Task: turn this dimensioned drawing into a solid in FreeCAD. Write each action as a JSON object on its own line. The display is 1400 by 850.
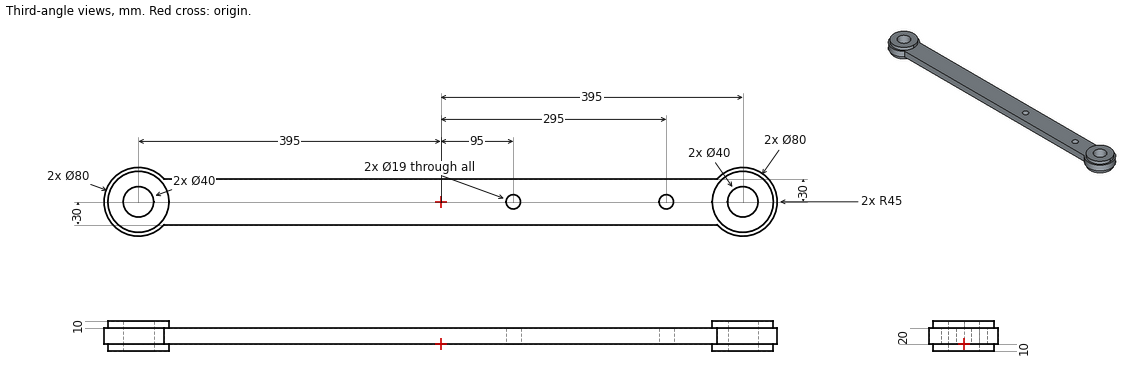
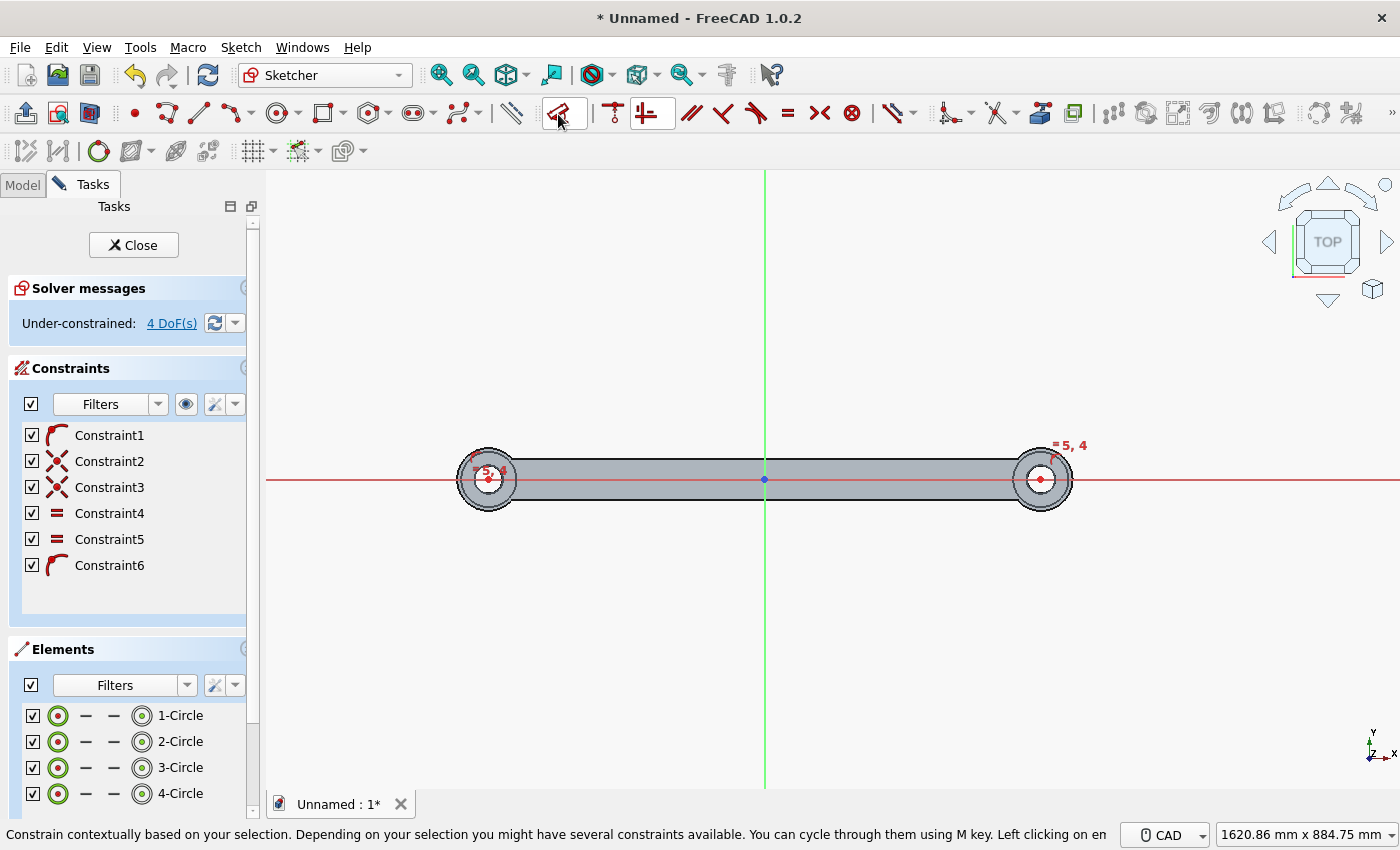
{"action": "left_click", "coordinate": [508, 460]}
{"action": "left_click", "coordinate": [530, 437]}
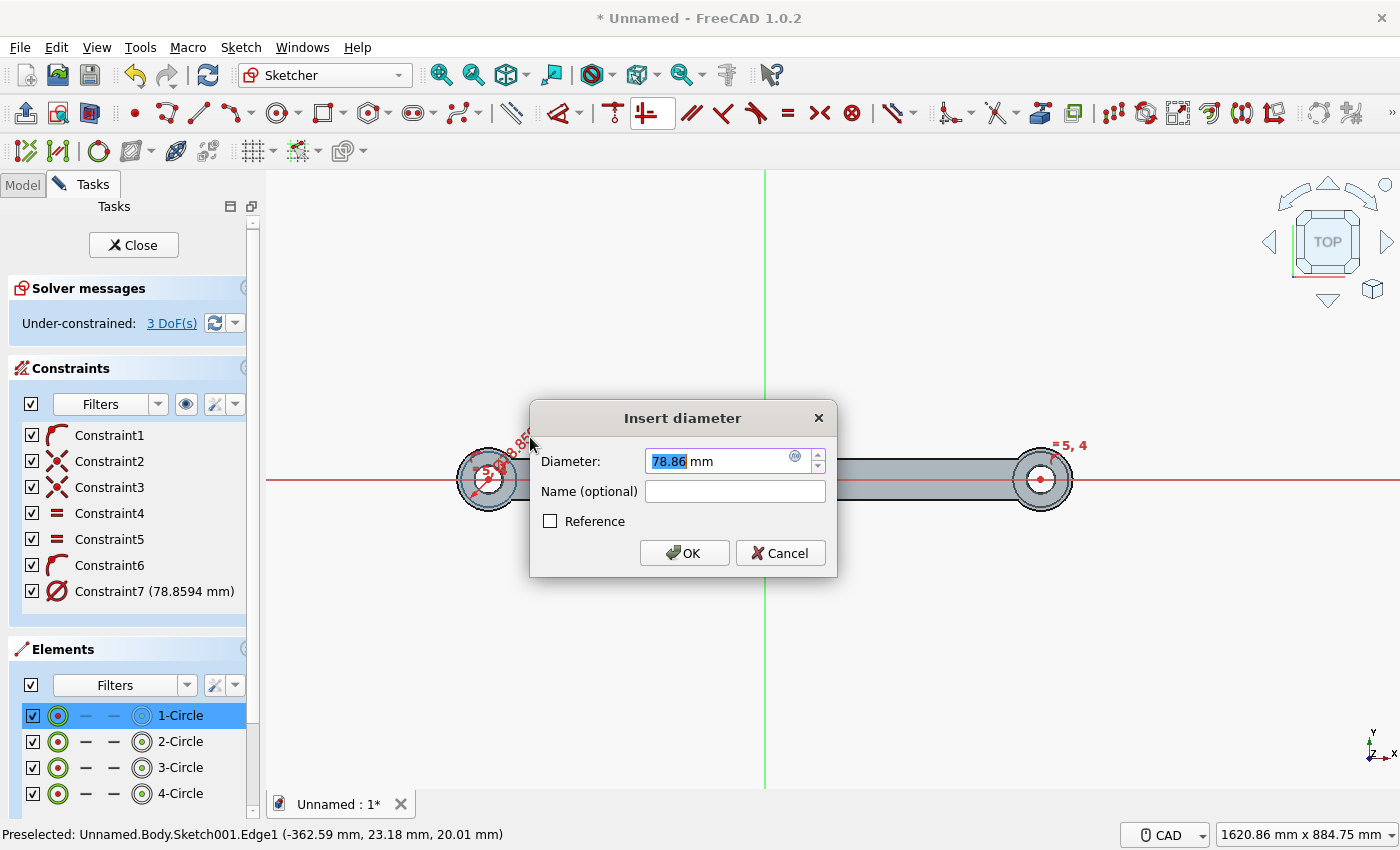
{"action": "type", "text": "80"}
{"action": "key", "text": "Return"}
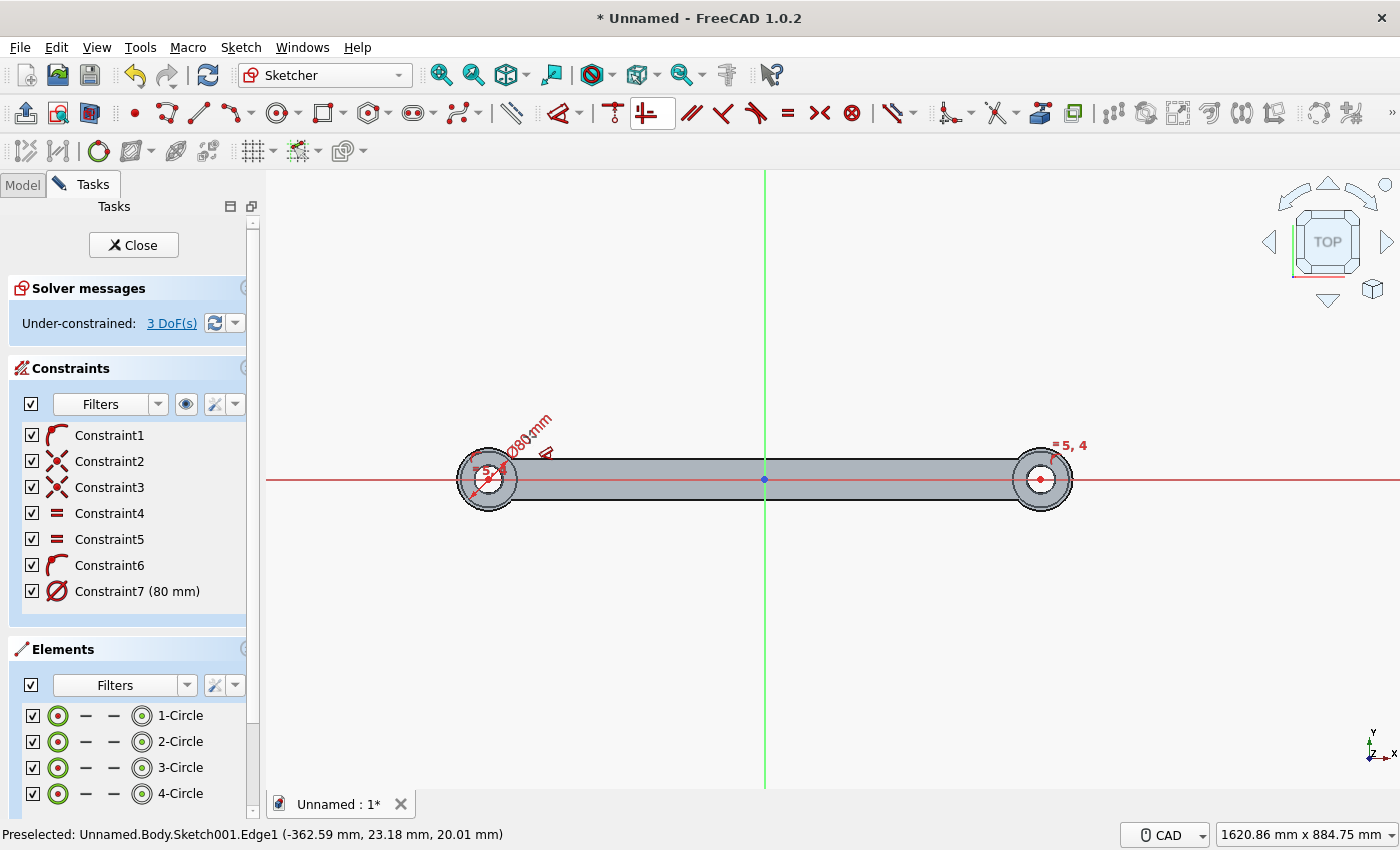
{"action": "scroll", "coordinate": [499, 469], "scroll_direction": "up", "scroll_amount": 2}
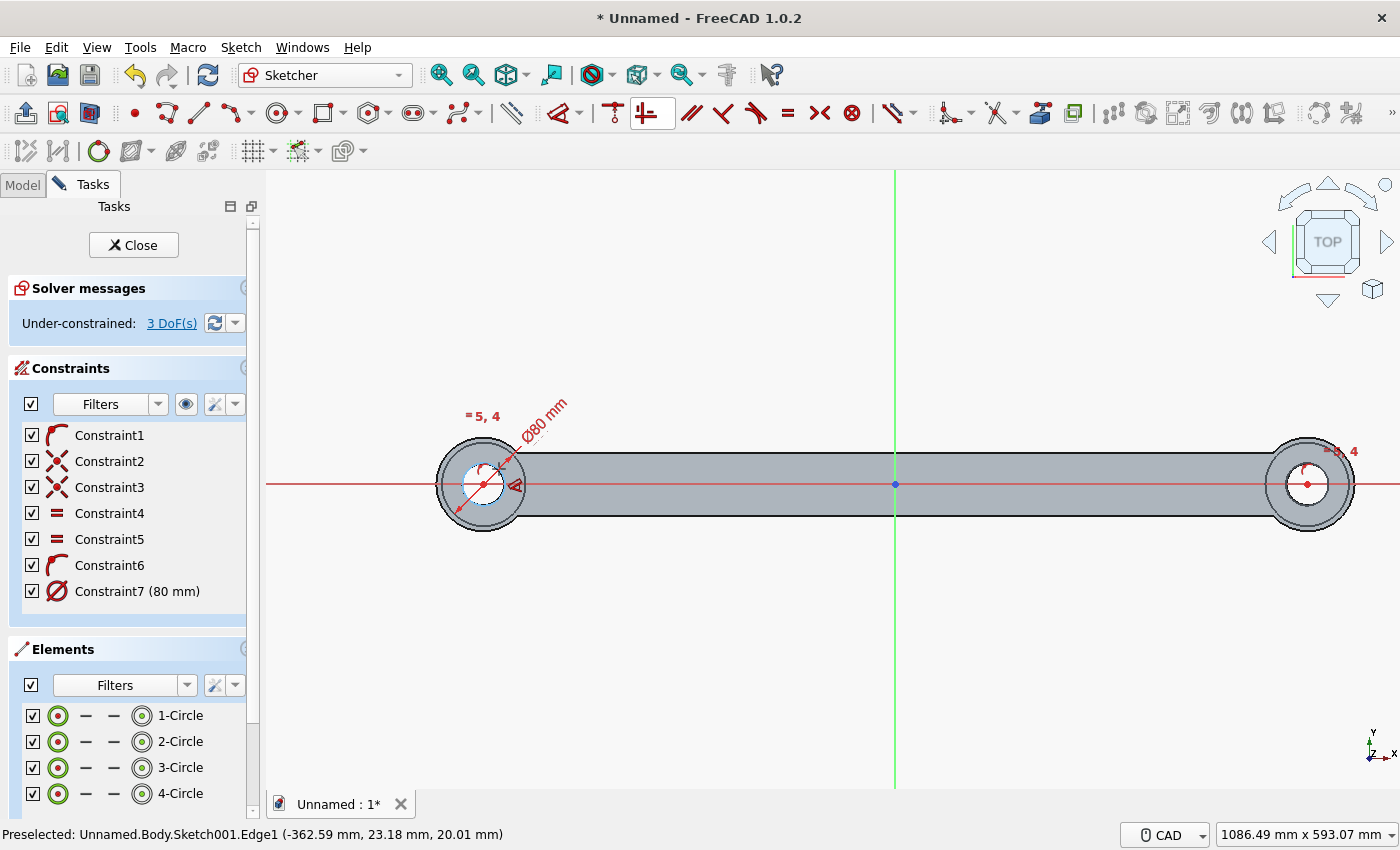
{"action": "left_click", "coordinate": [499, 469]}
{"action": "left_click", "coordinate": [557, 463]}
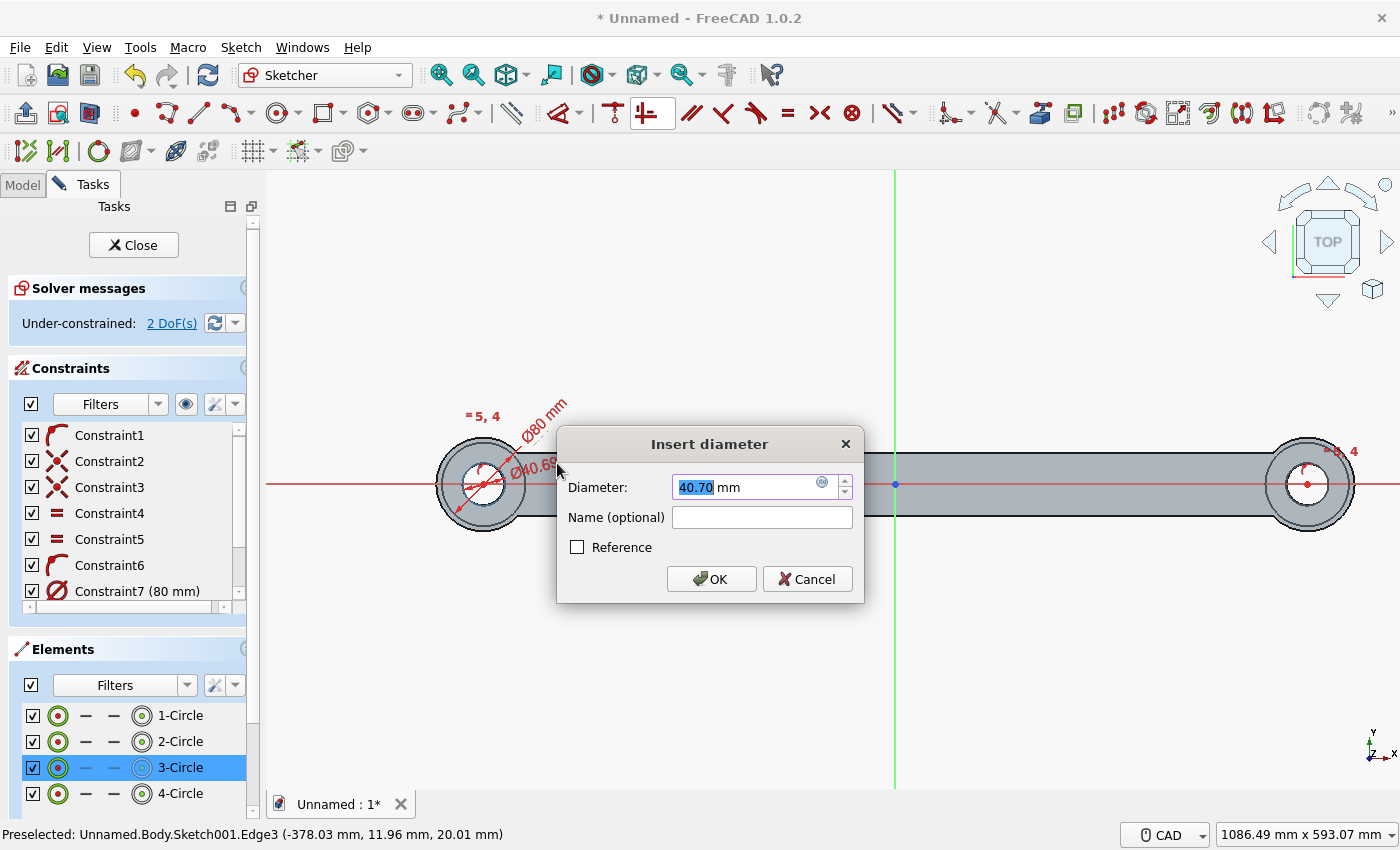
{"action": "type", "text": "40"}
{"action": "key", "text": "Return"}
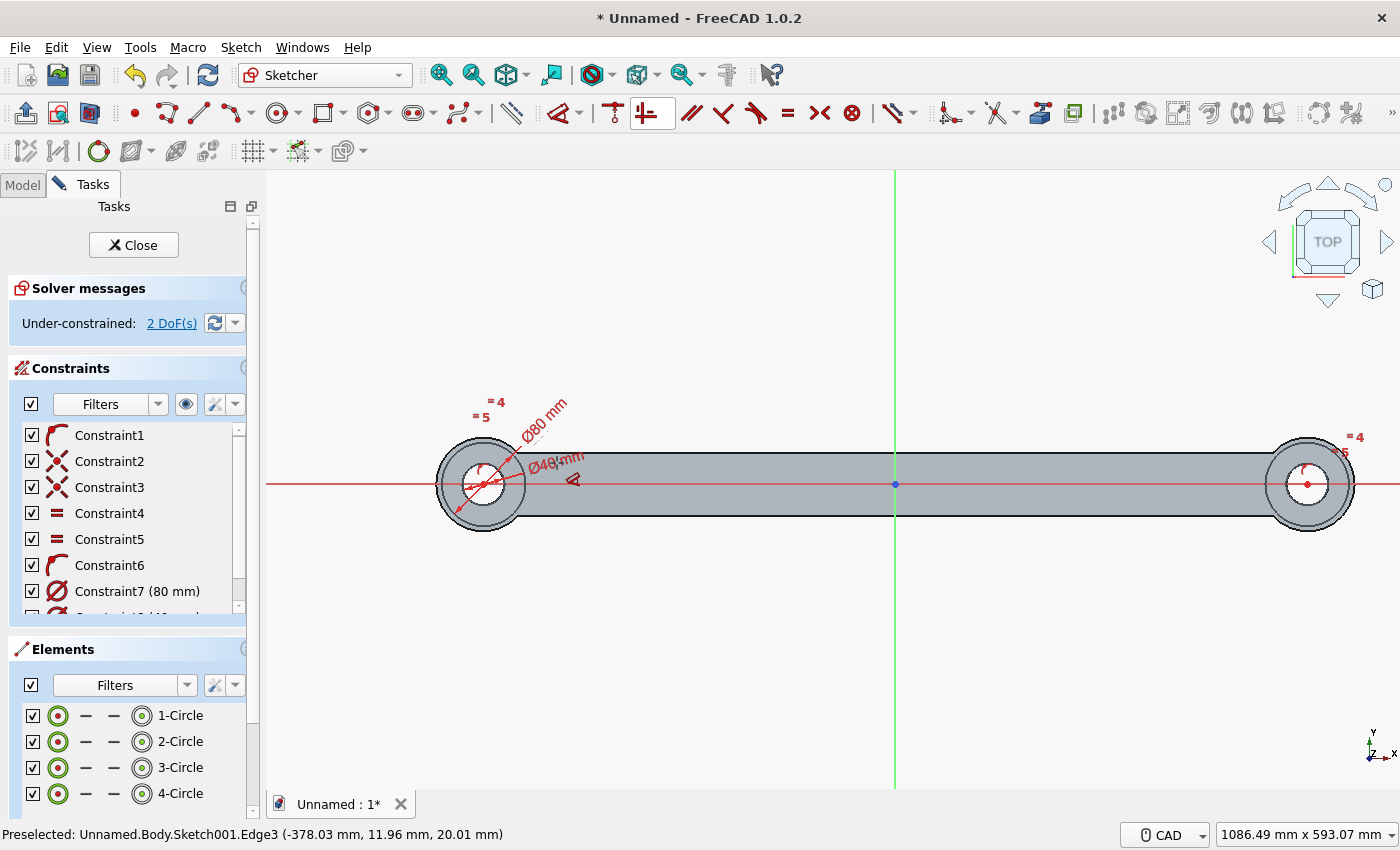
{"action": "left_click", "coordinate": [484, 484]}
{"action": "left_click", "coordinate": [690, 518]}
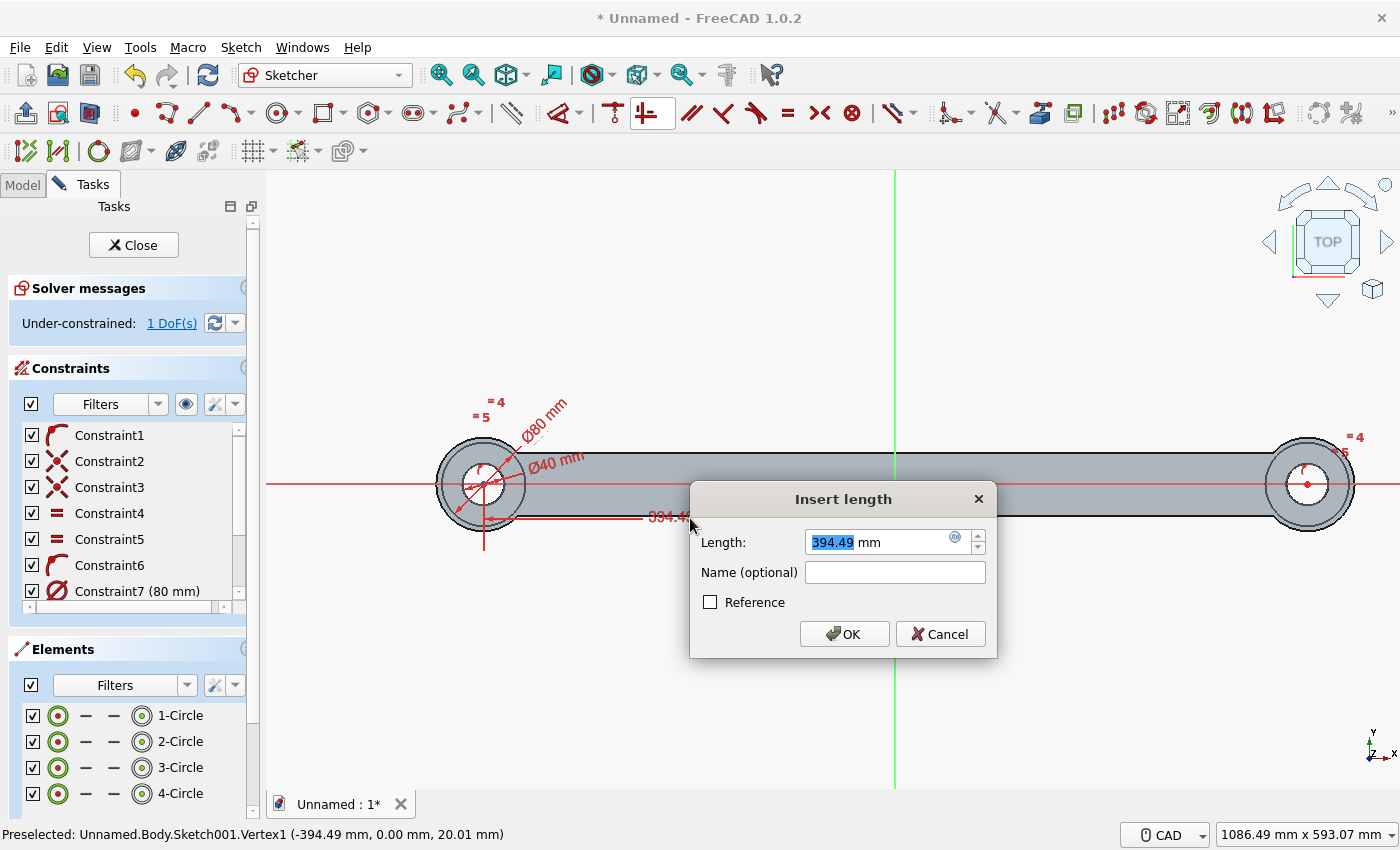
{"action": "type", "text": "395"}
{"action": "key", "text": "Return"}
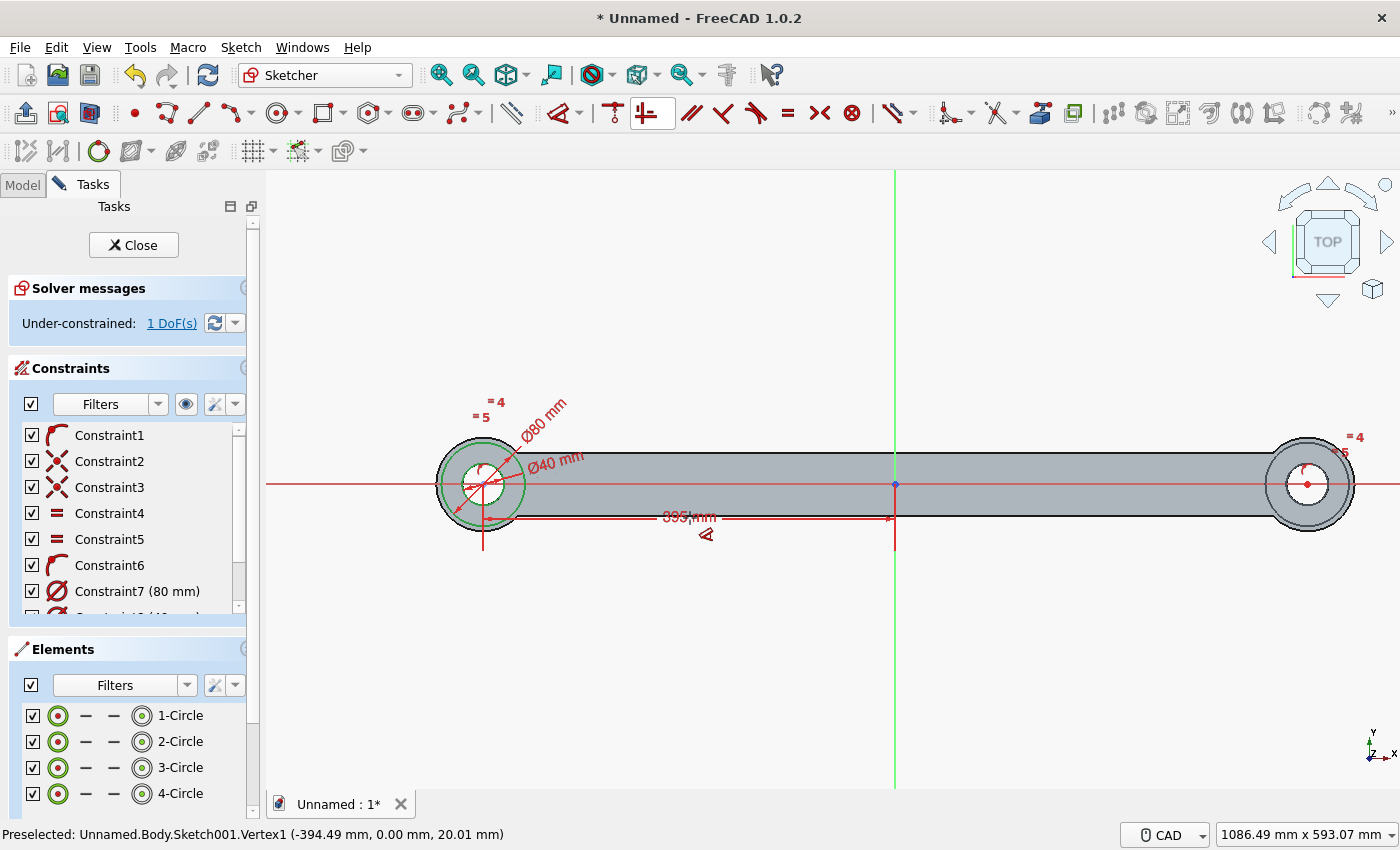
{"action": "scroll", "coordinate": [498, 469], "scroll_direction": "down", "scroll_amount": 2}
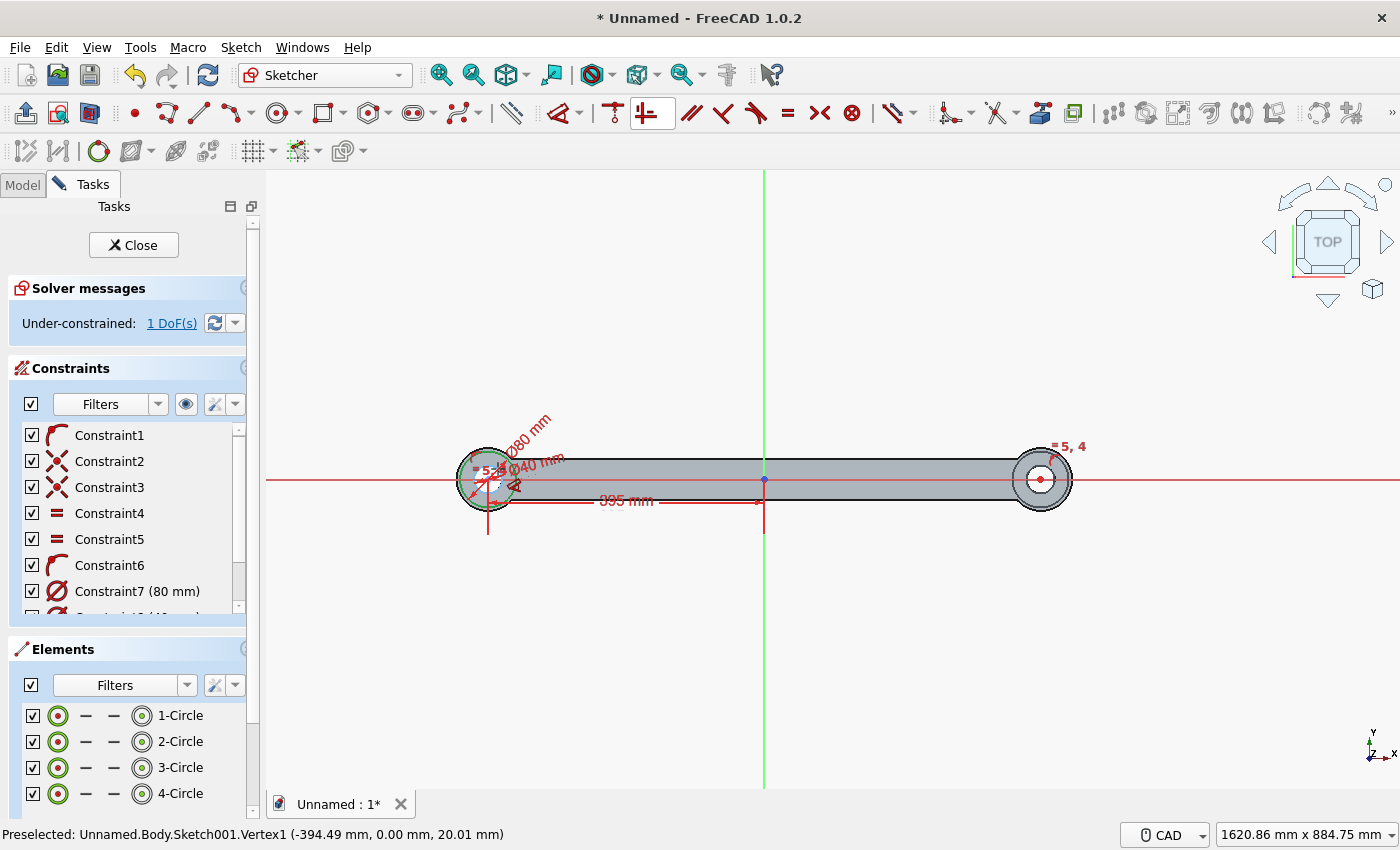
{"action": "left_click", "coordinate": [1040, 480]}
{"action": "left_click", "coordinate": [902, 514]}